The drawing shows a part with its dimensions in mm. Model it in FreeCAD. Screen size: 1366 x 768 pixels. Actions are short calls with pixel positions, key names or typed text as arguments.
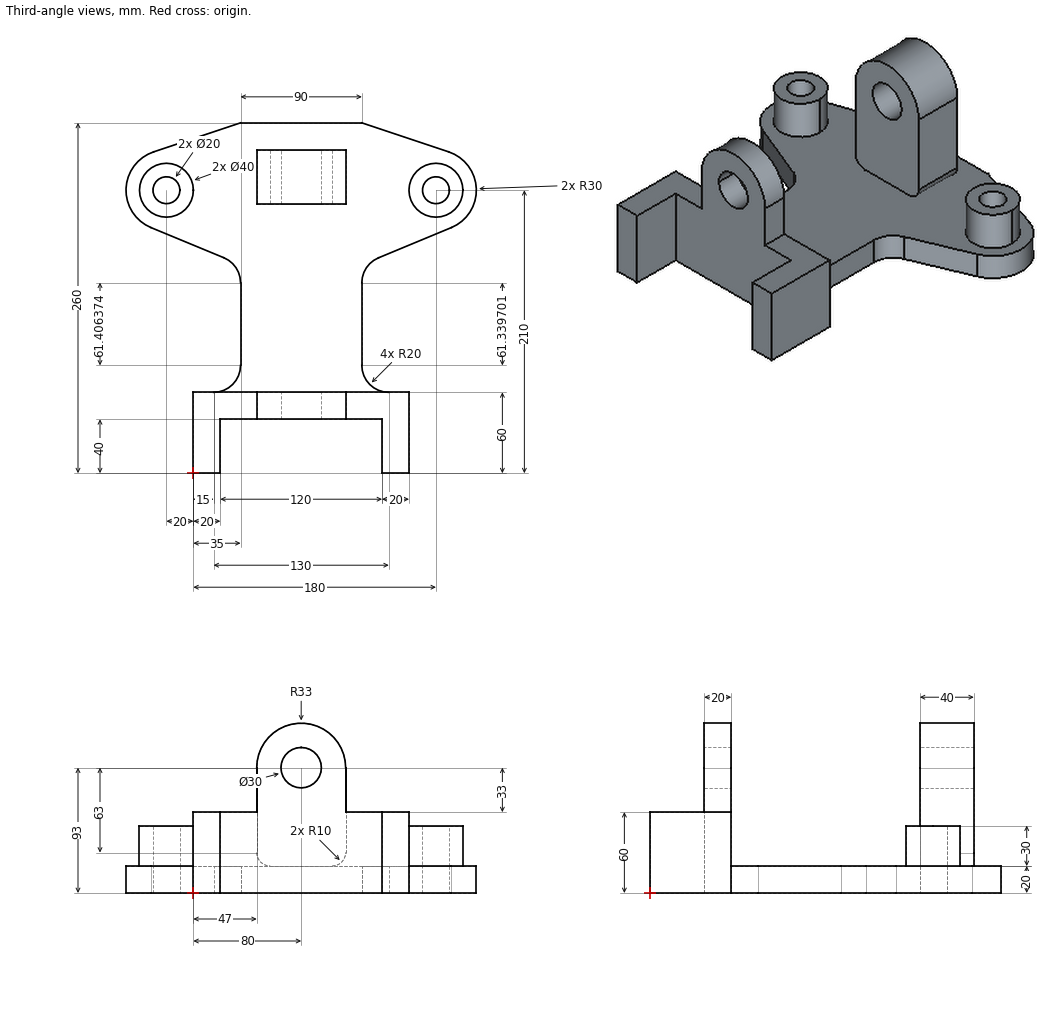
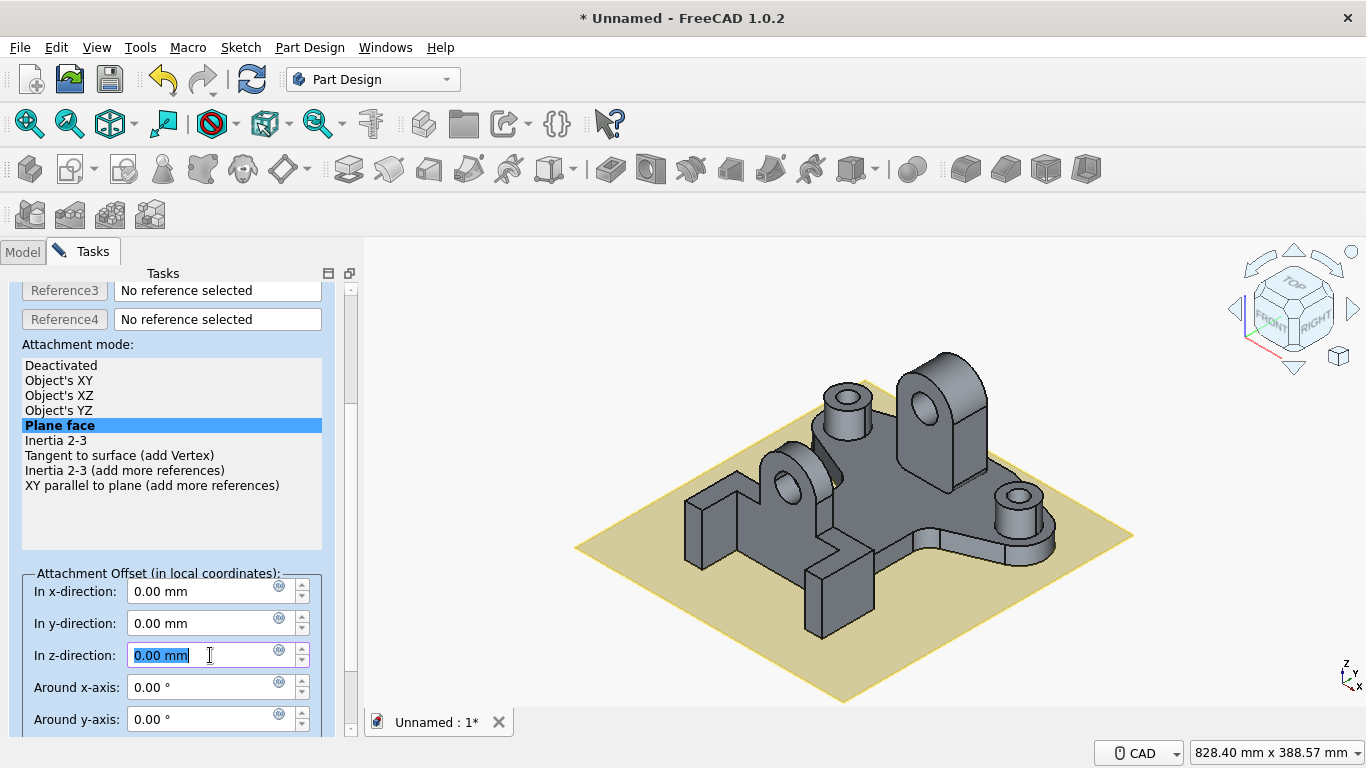
text(-20)
key(Tab)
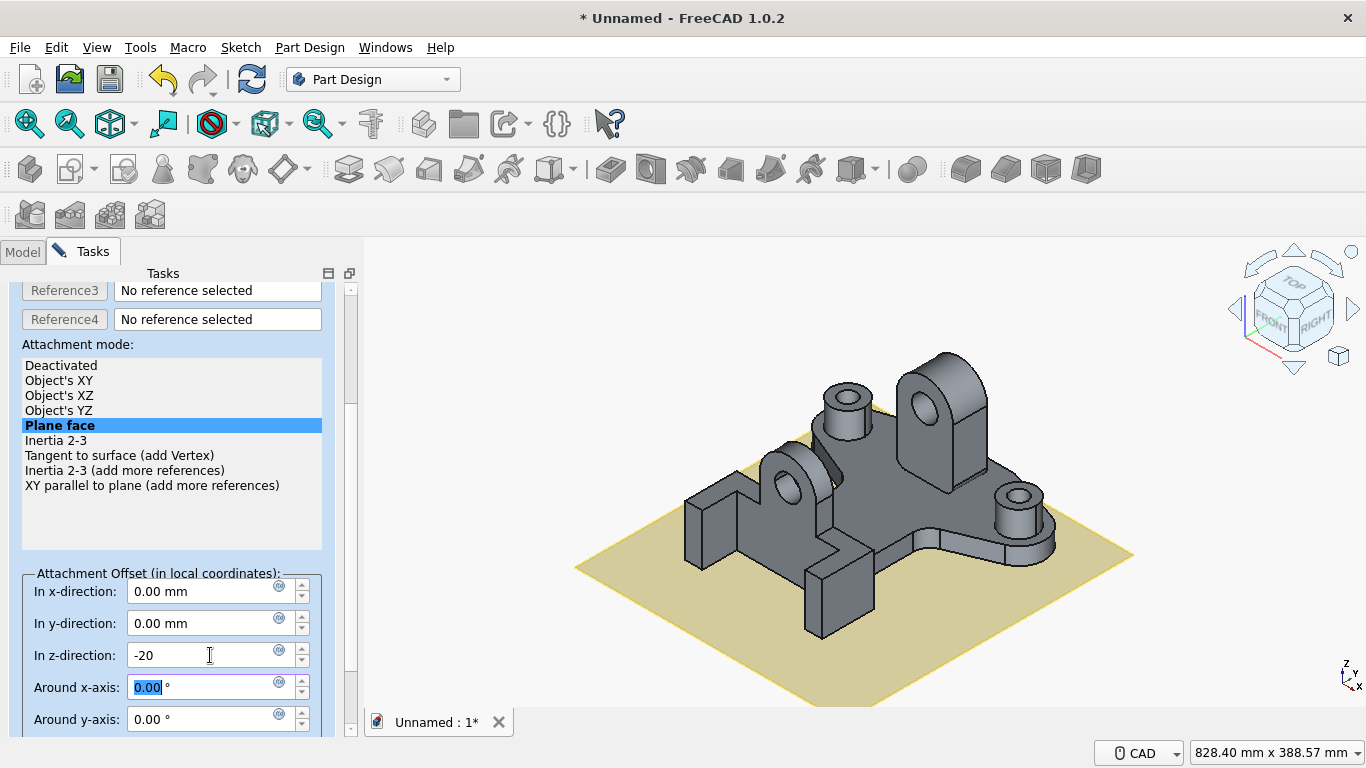
scroll(351, 510, up, 4)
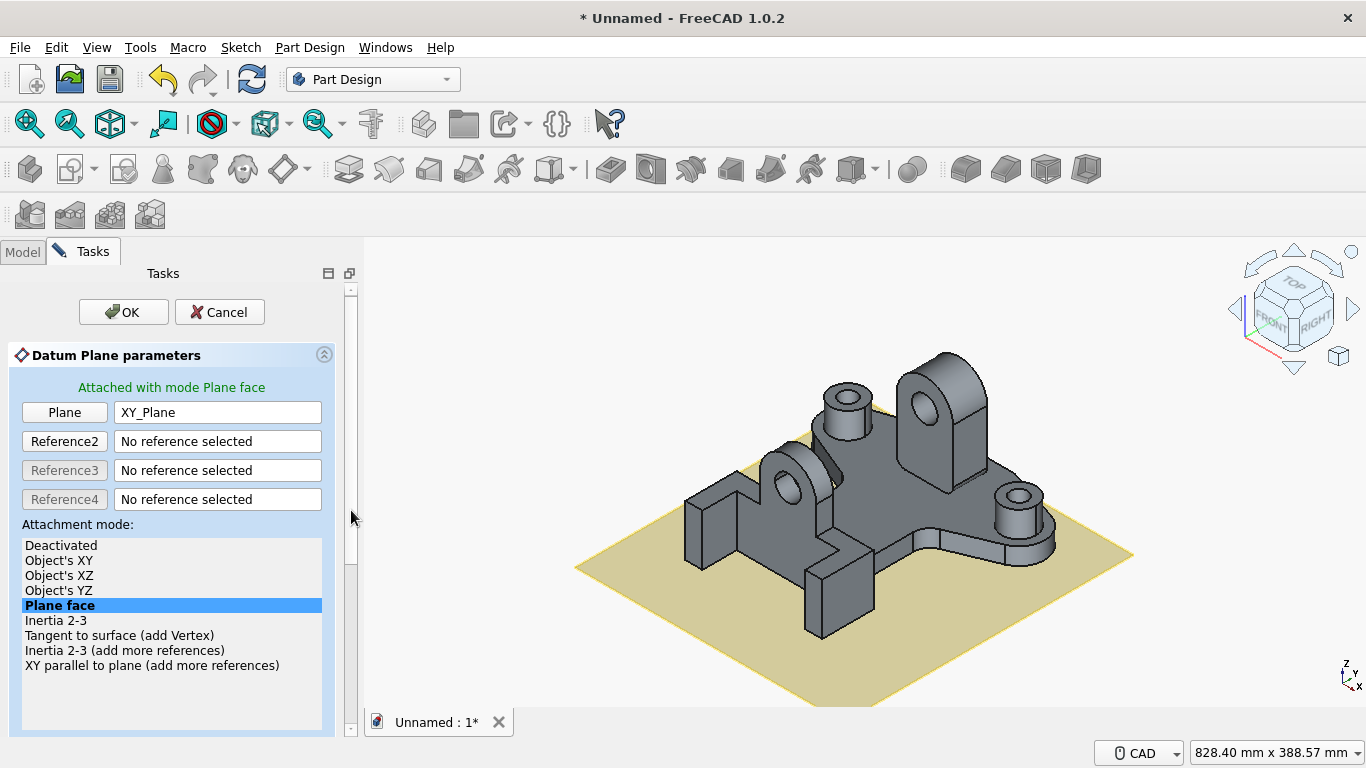
click(124, 312)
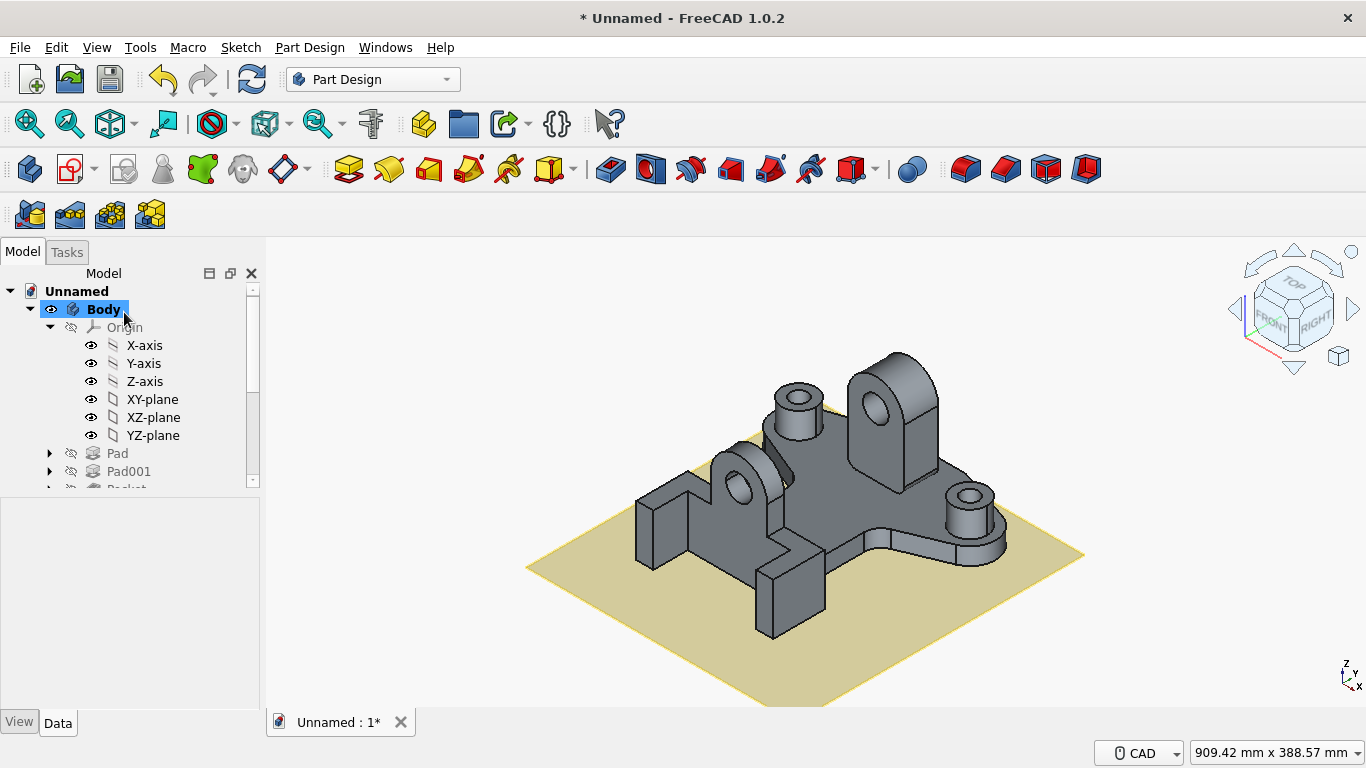
scroll(100, 377, down, 3)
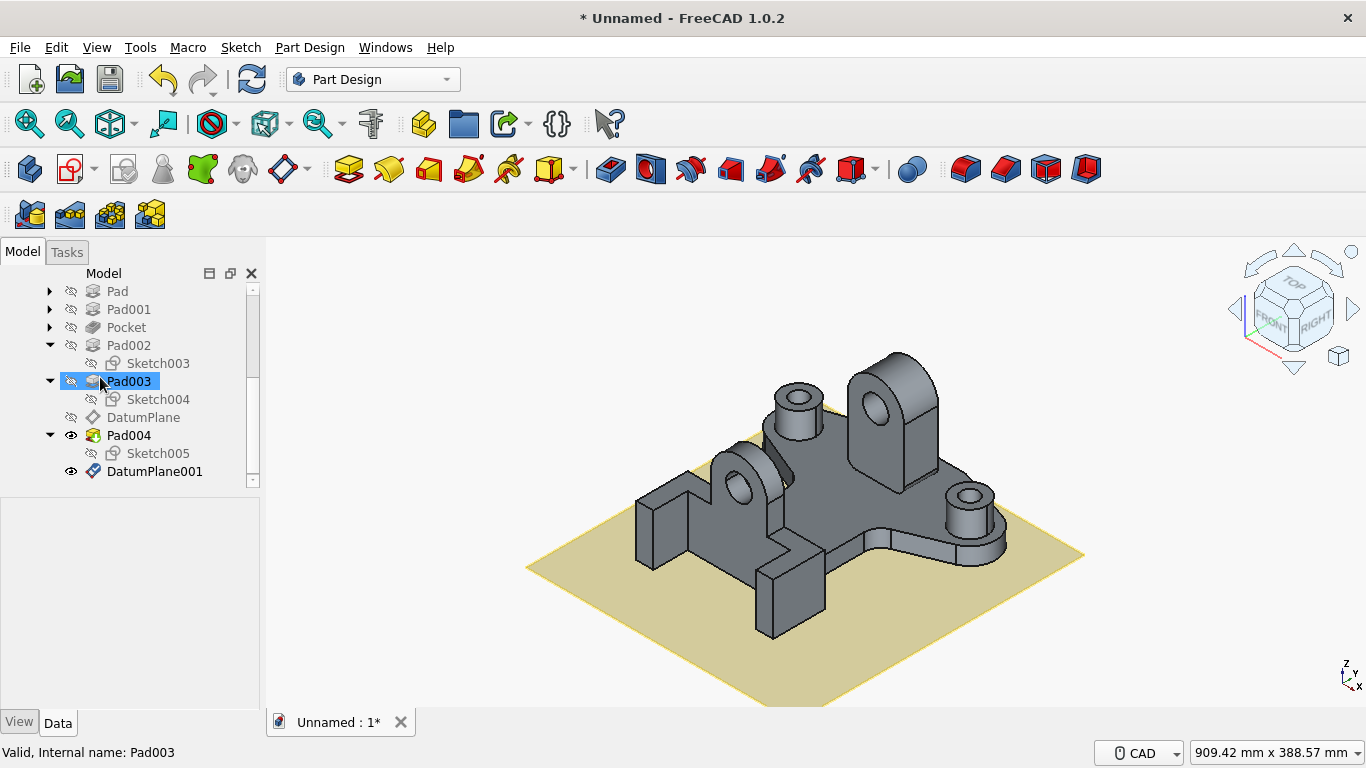
click(116, 471)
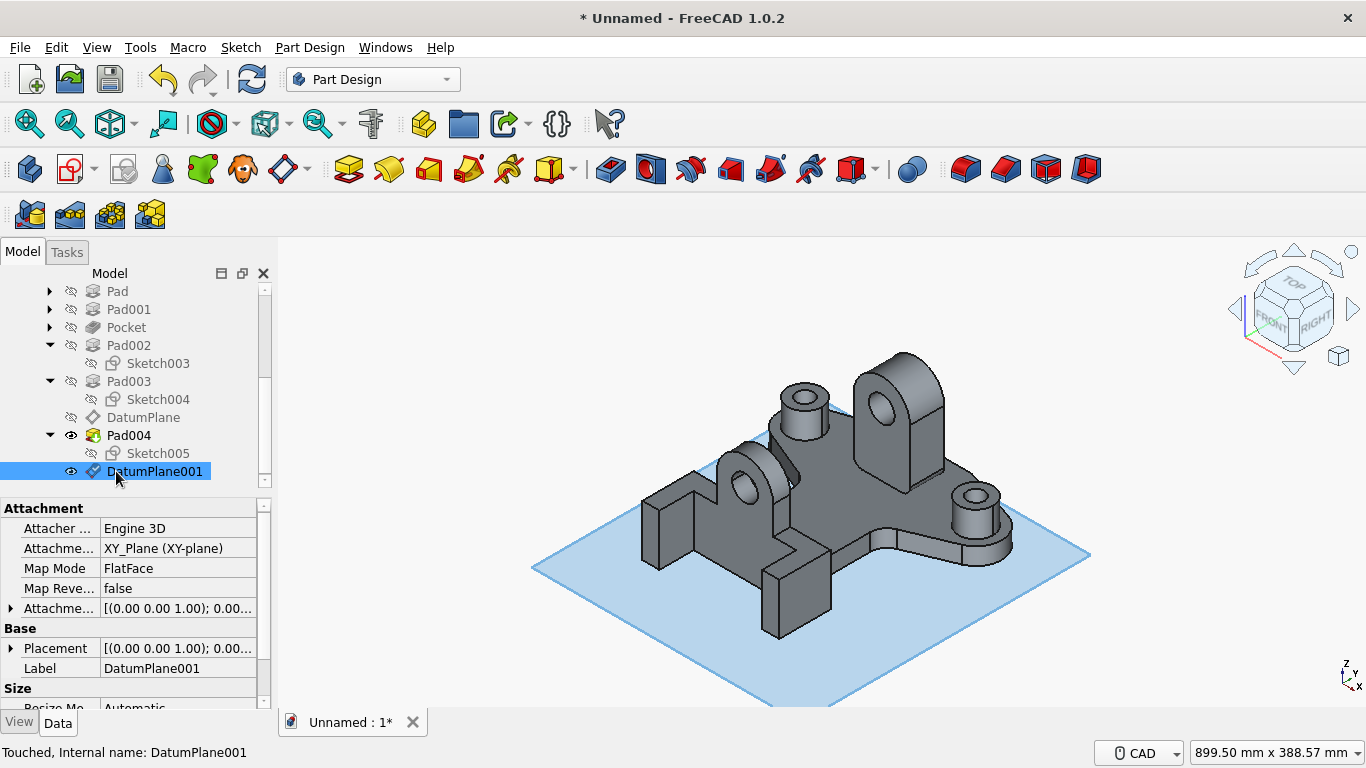
click(70, 170)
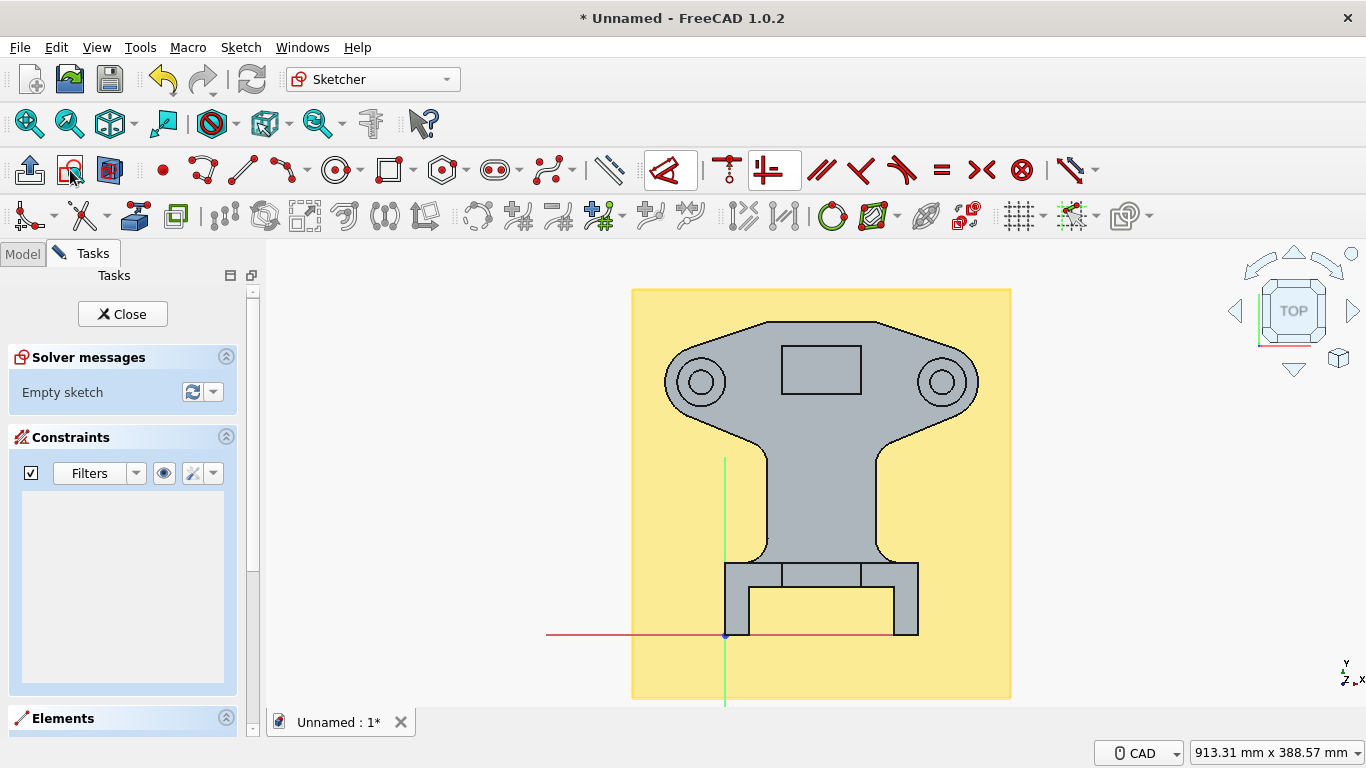
click(110, 170)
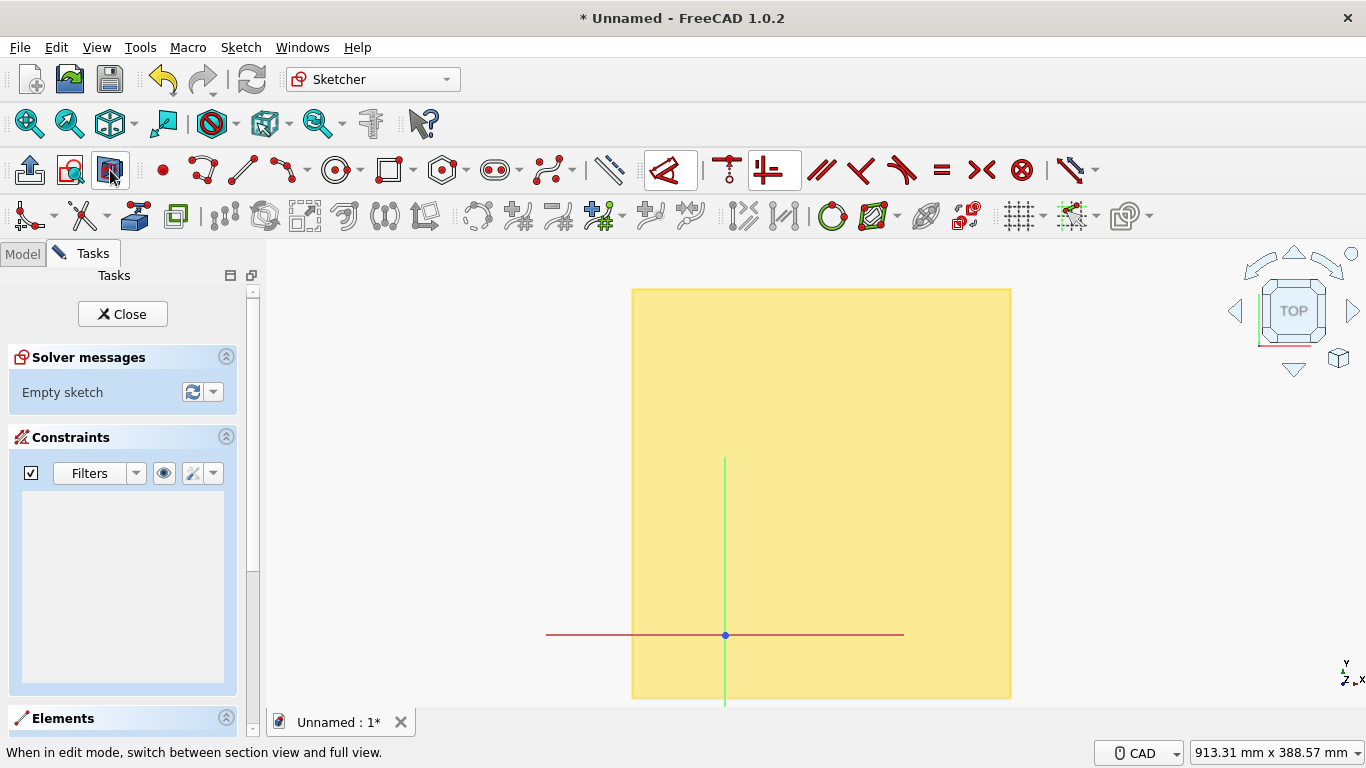
click(336, 170)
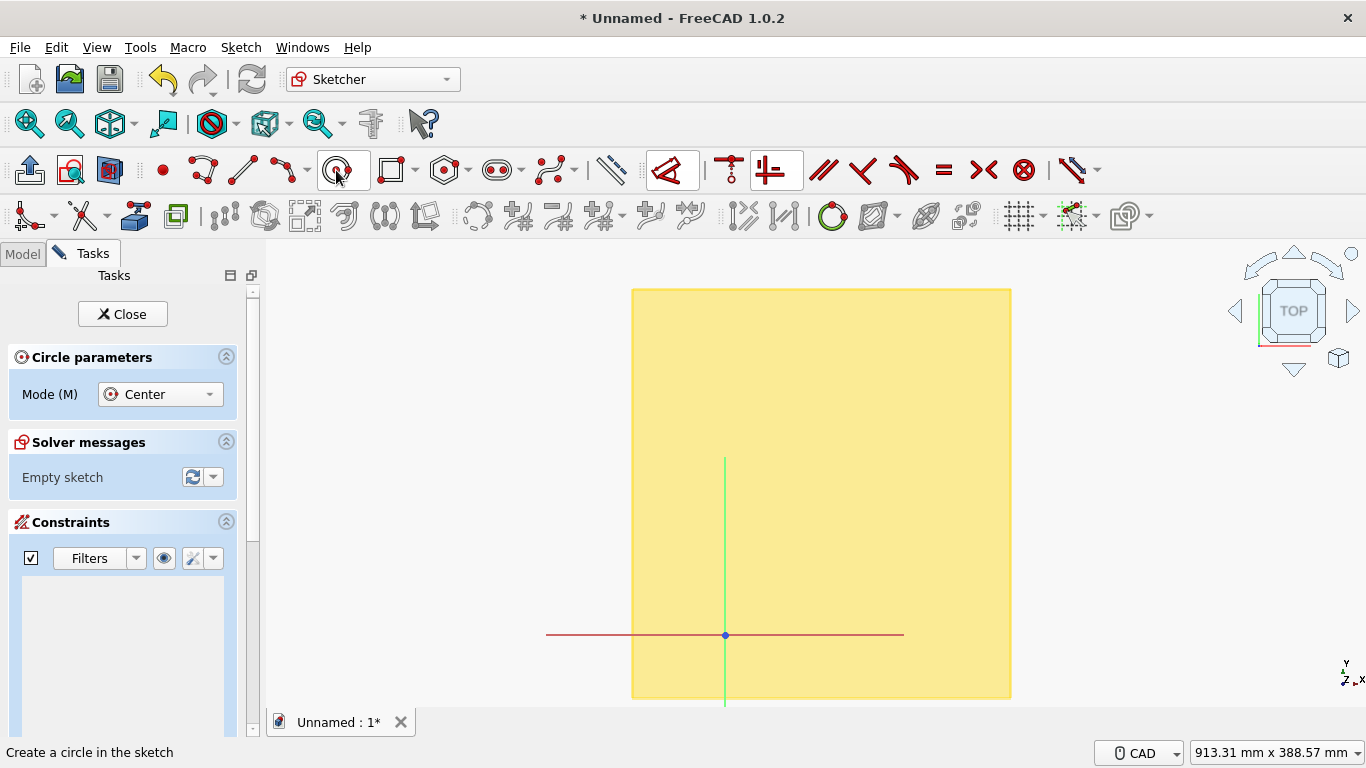
scroll(701, 382, up, 4)